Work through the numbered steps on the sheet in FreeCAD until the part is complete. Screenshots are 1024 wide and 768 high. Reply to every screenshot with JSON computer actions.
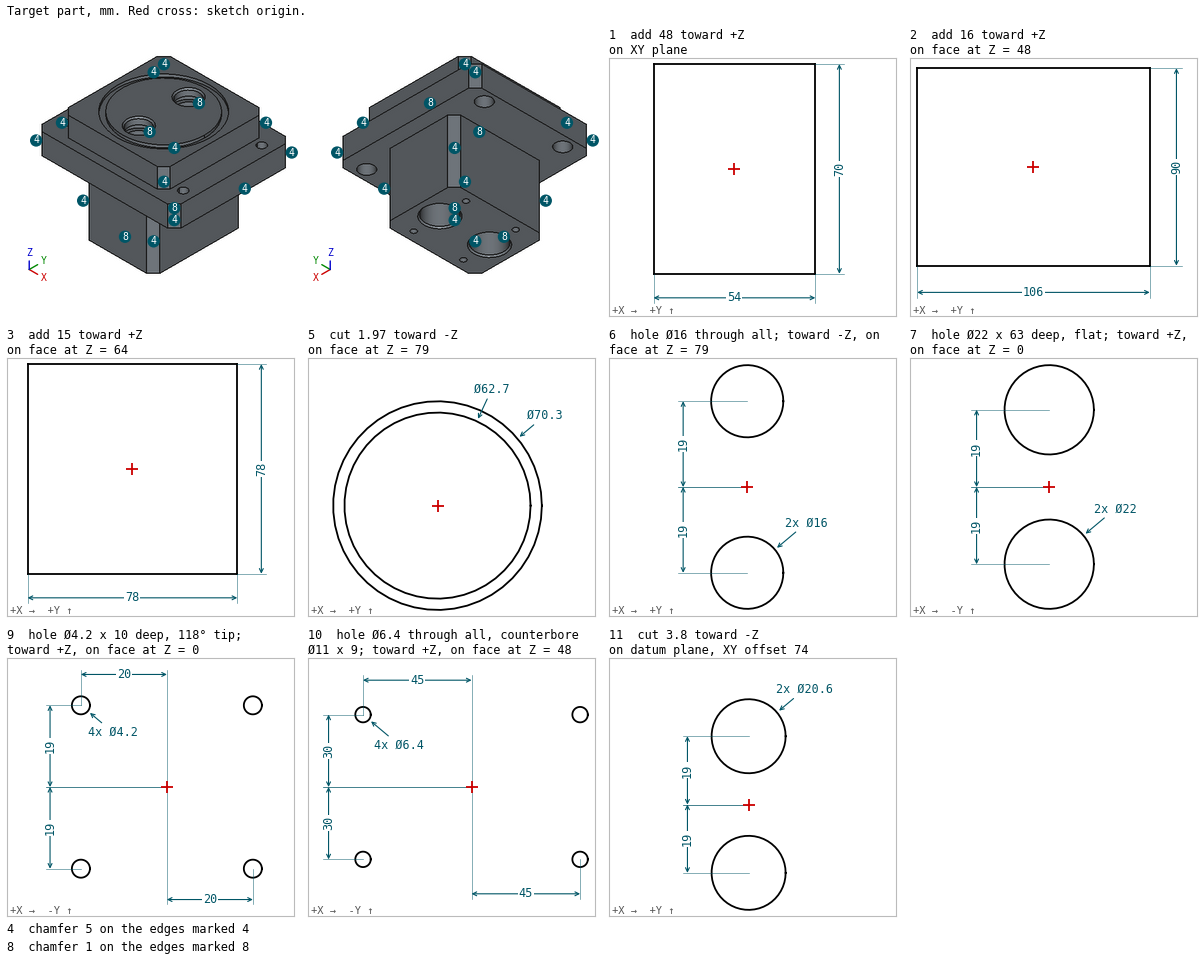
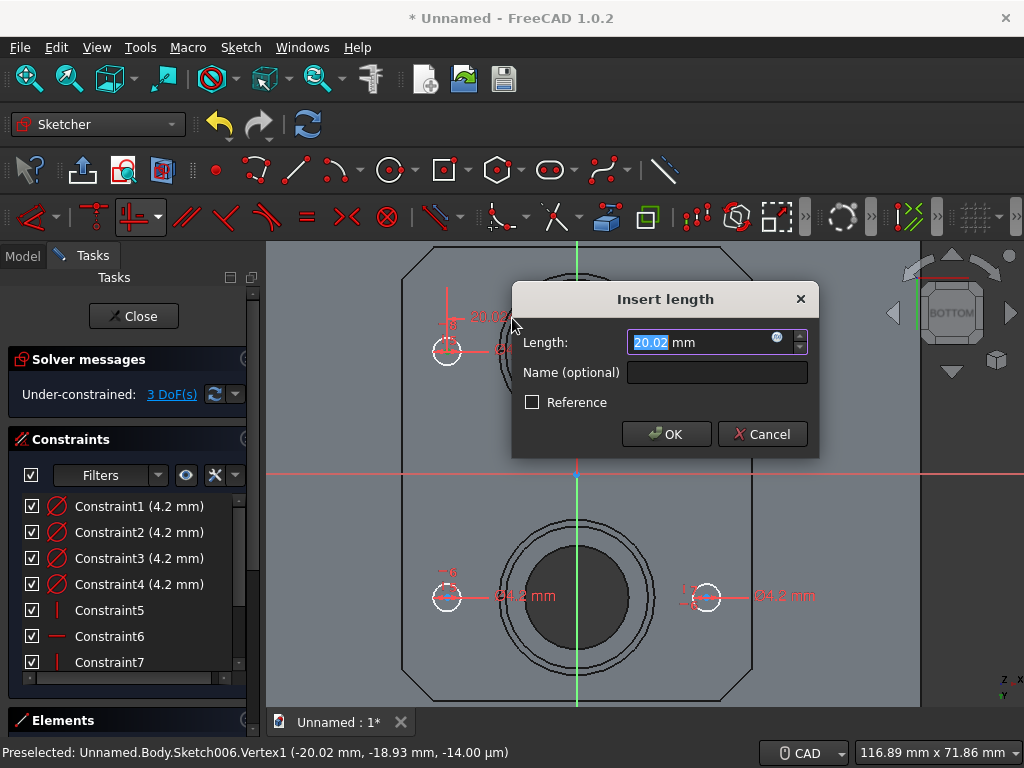
{"action": "type", "text": "20"}
{"action": "key", "text": "Return"}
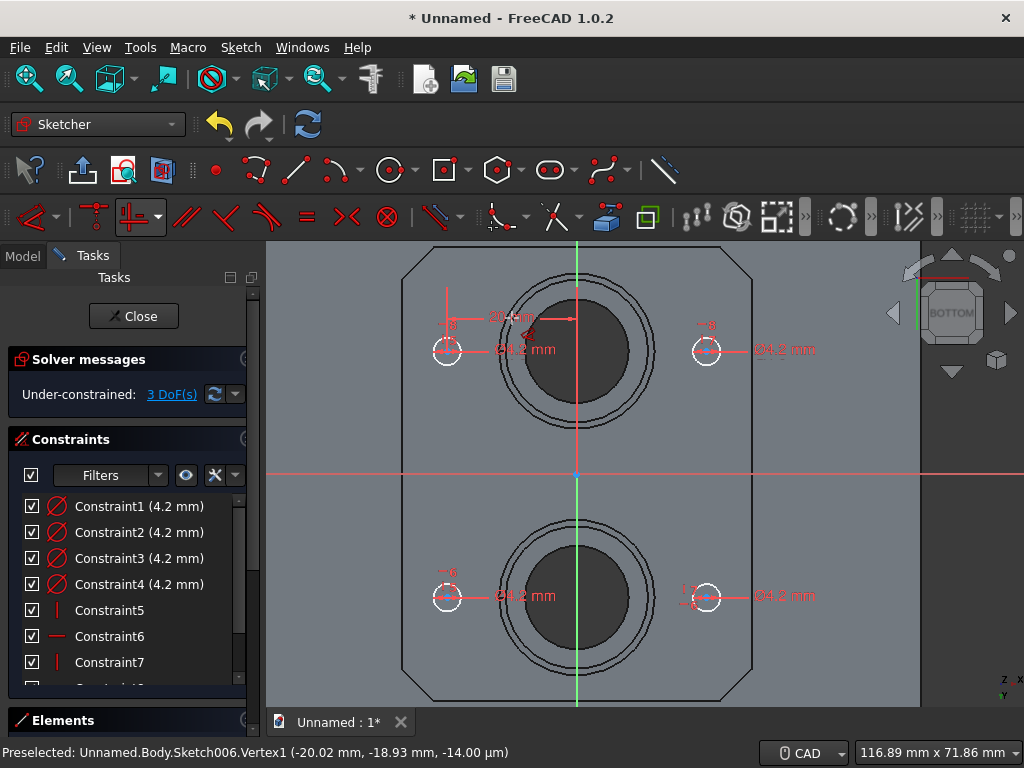
{"action": "left_click", "coordinate": [447, 352]}
{"action": "left_click", "coordinate": [413, 413]}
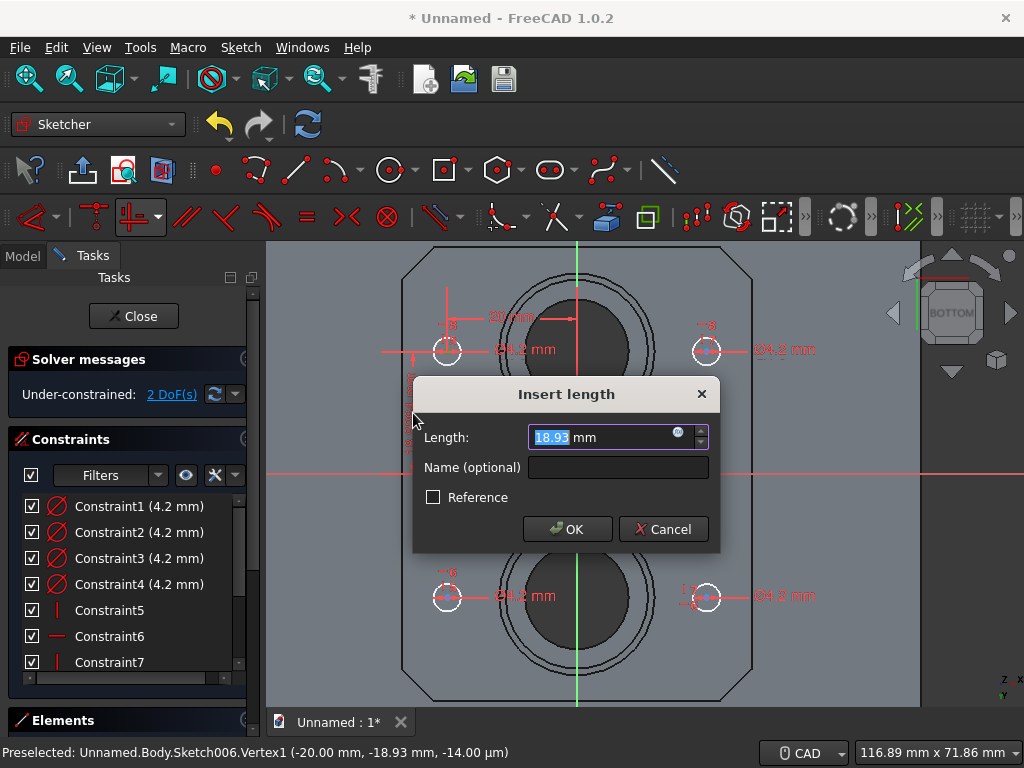
{"action": "type", "text": "19"}
{"action": "key", "text": "Return"}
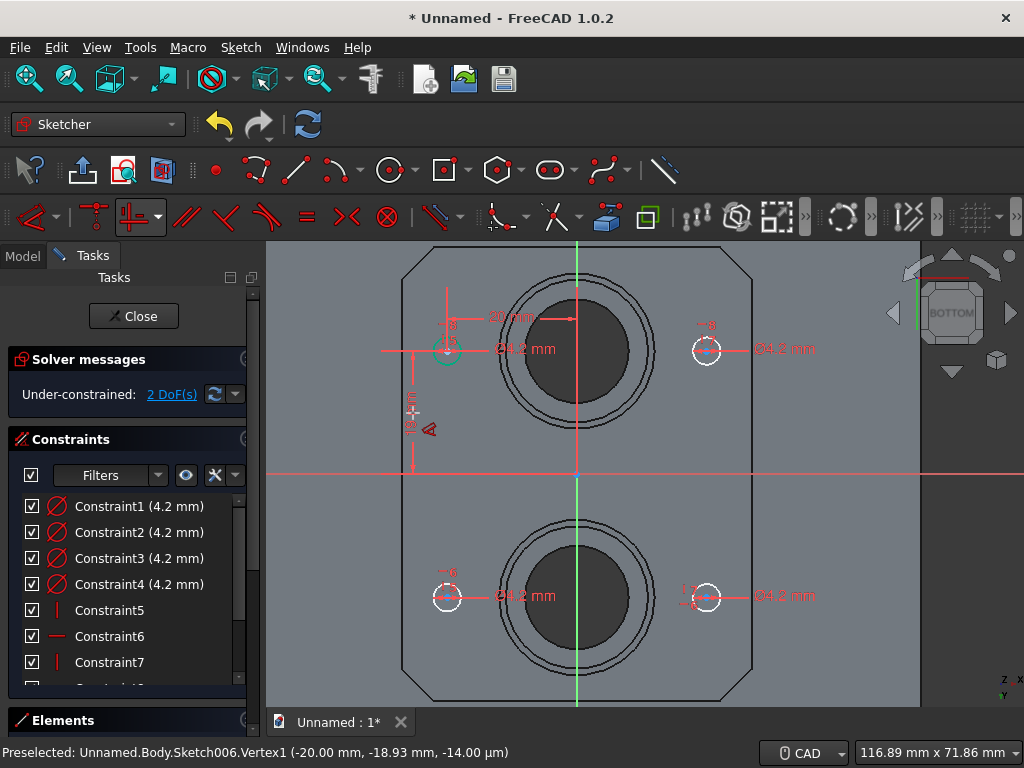
{"action": "left_click", "coordinate": [447, 598]}
{"action": "left_click", "coordinate": [413, 536]}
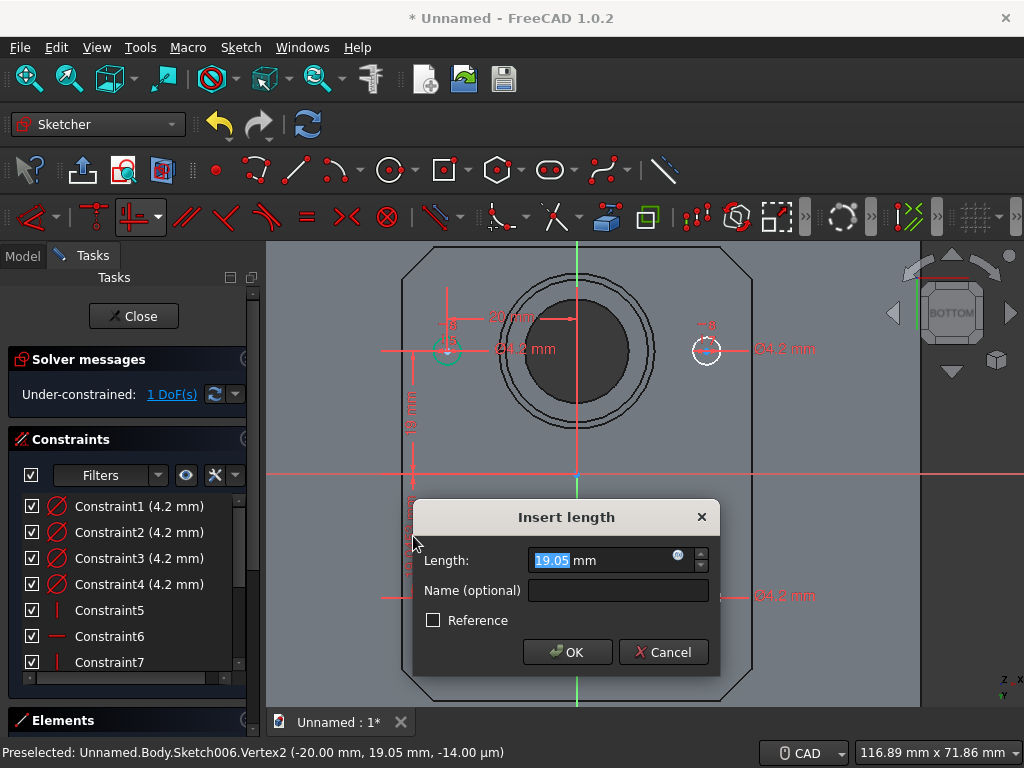
{"action": "type", "text": "19"}
{"action": "key", "text": "Return"}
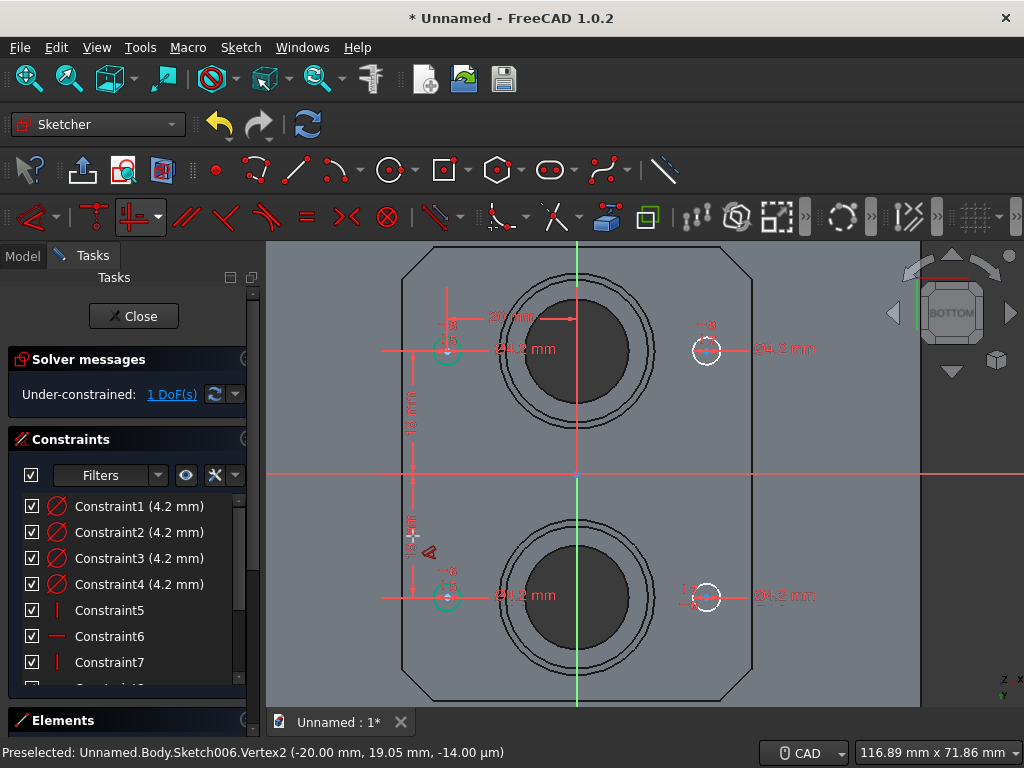
{"action": "left_click", "coordinate": [707, 598]}
{"action": "left_click", "coordinate": [642, 632]}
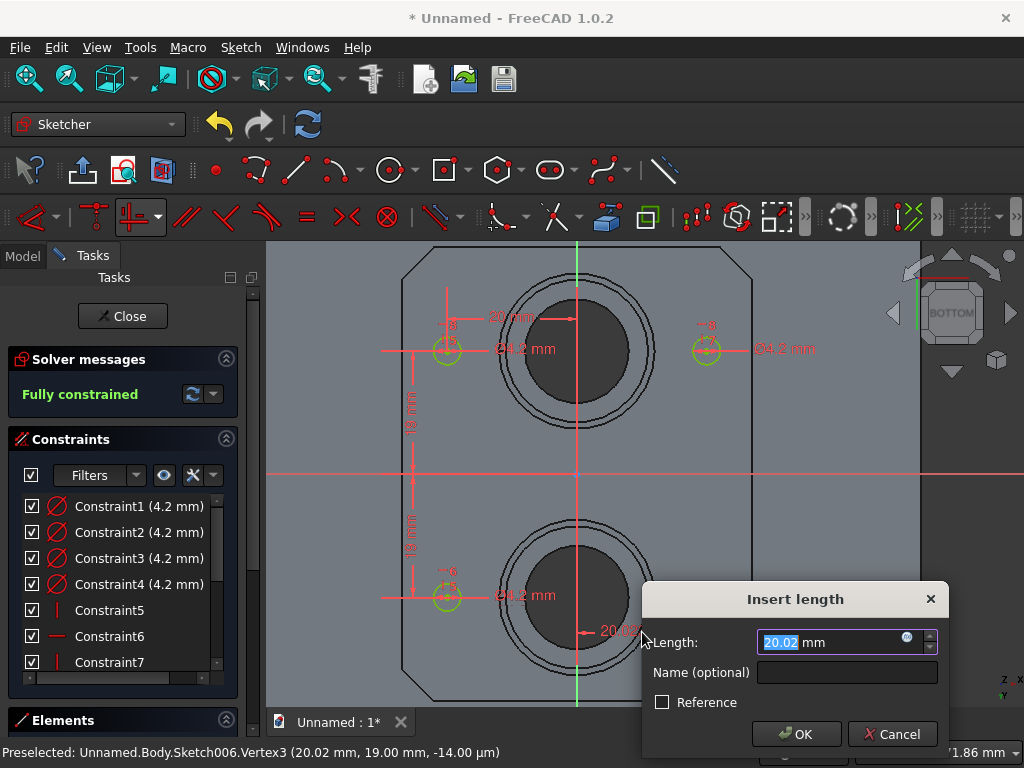
{"action": "type", "text": "20"}
{"action": "key", "text": "Return"}
{"action": "key", "text": "Escape"}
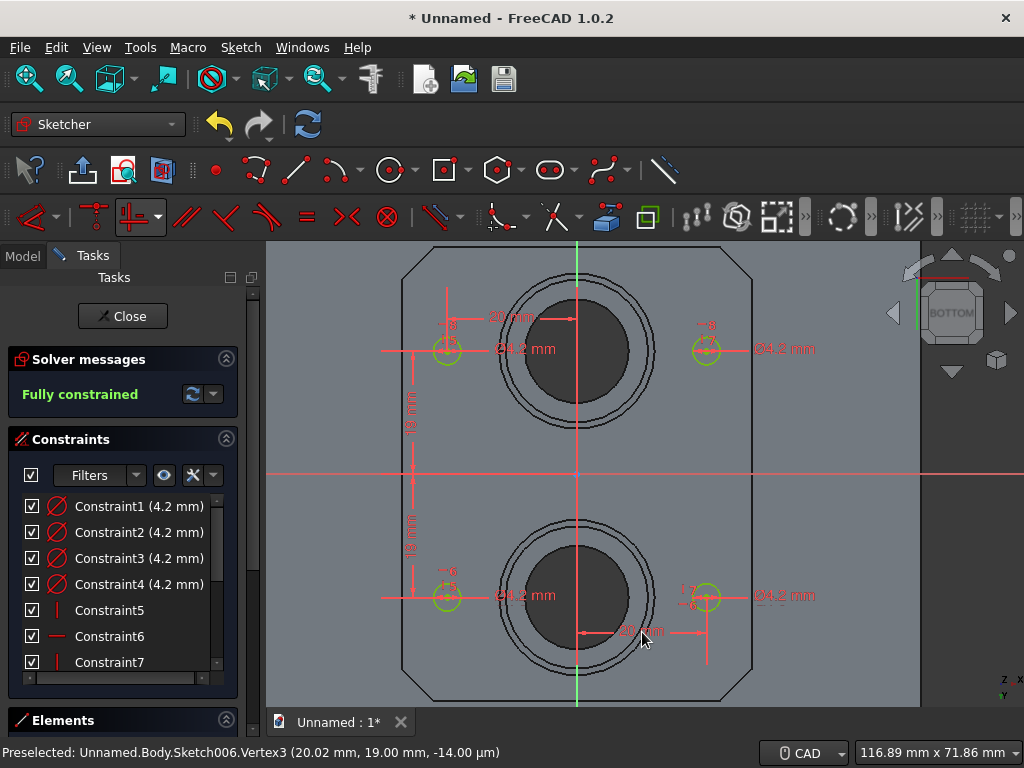
{"action": "left_click", "coordinate": [123, 316]}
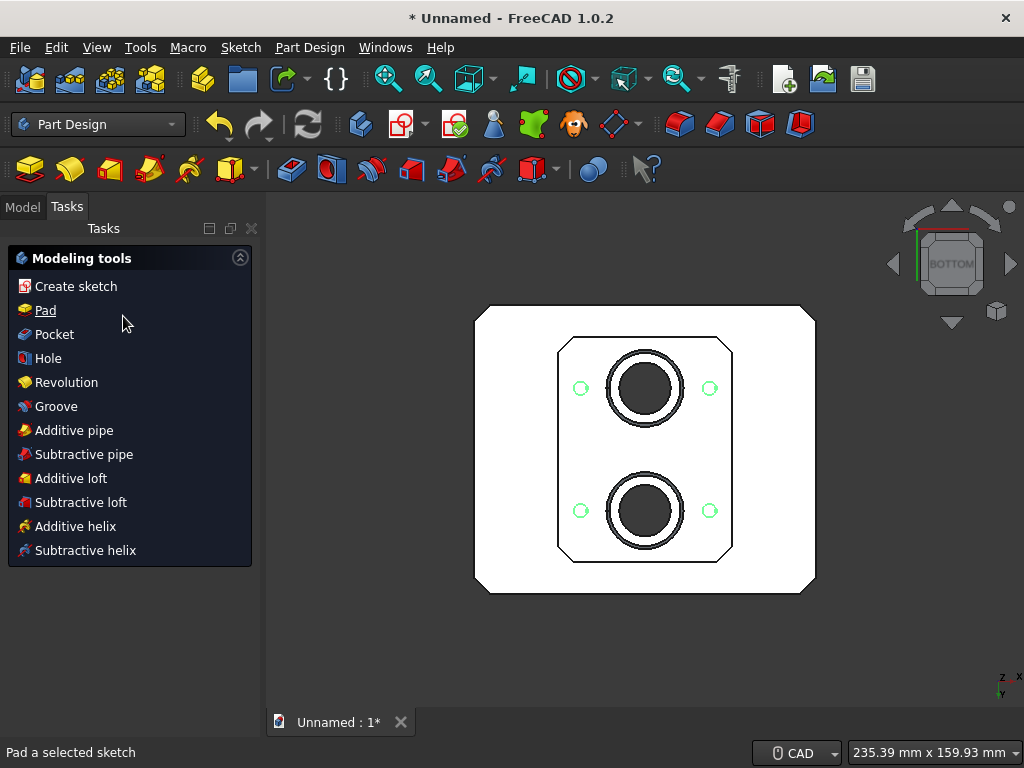
{"action": "left_click", "coordinate": [332, 170]}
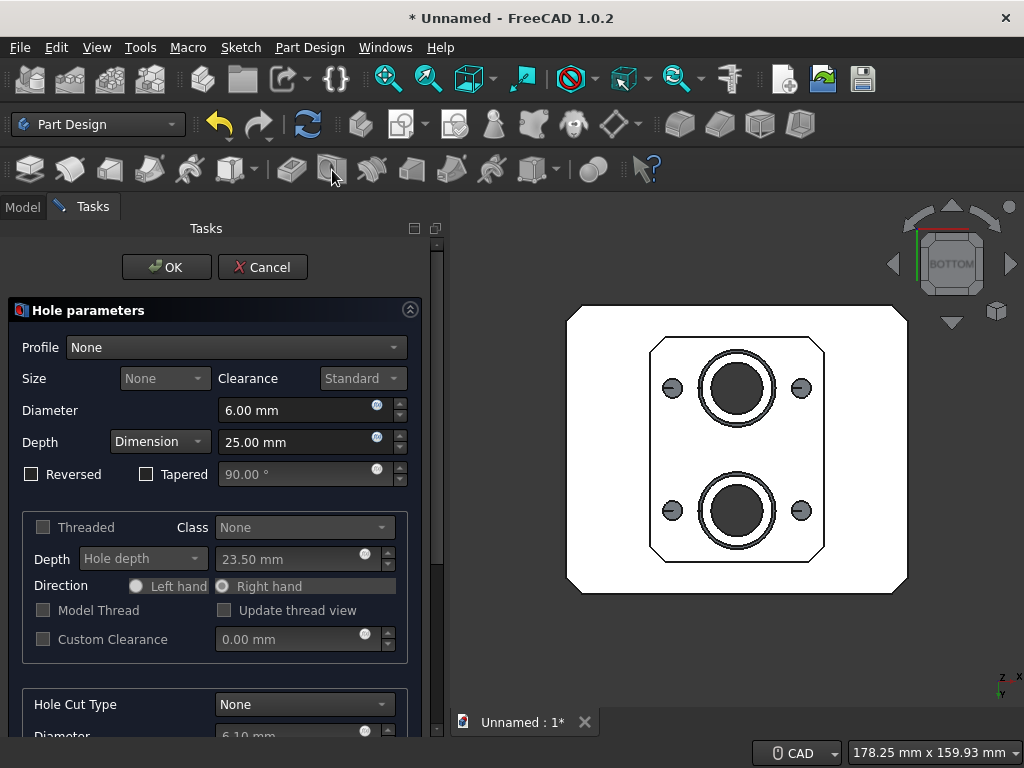
{"action": "triple_click", "coordinate": [305, 410]}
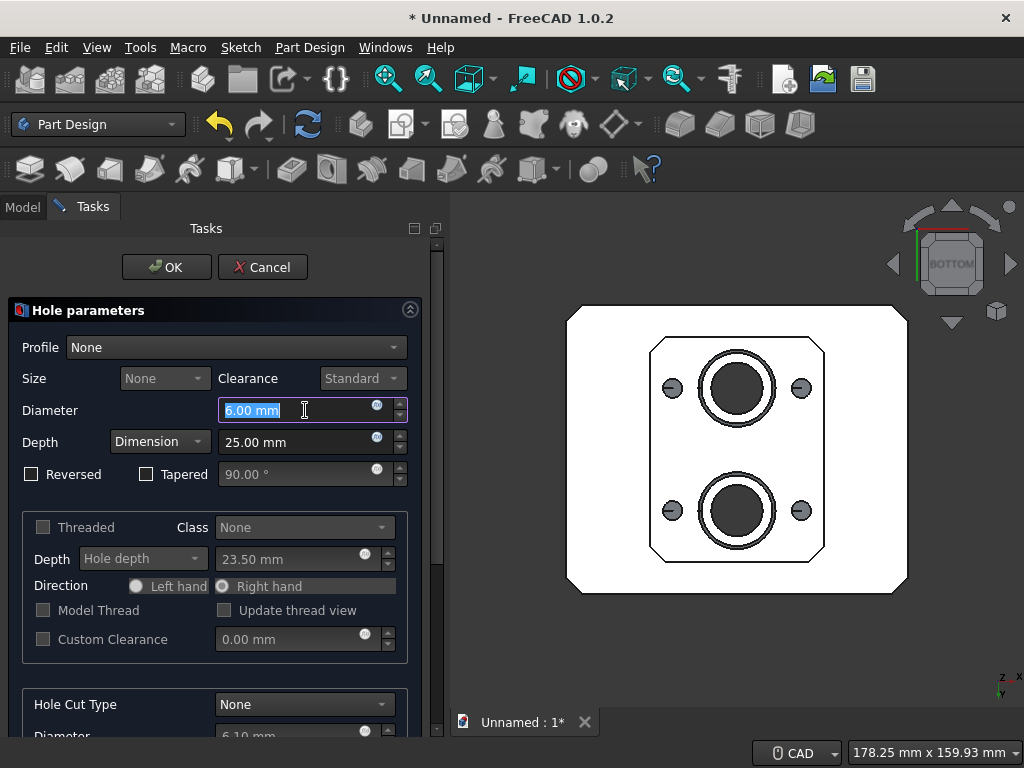
{"action": "type", "text": "4.2"}
{"action": "key", "text": "Tab"}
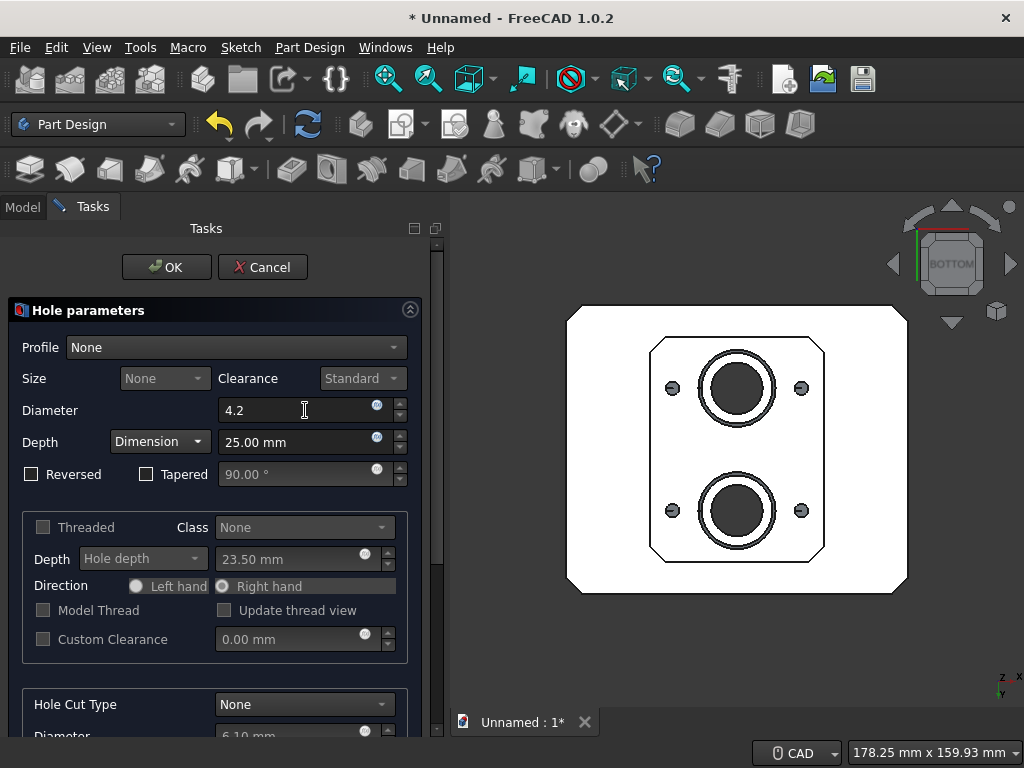
{"action": "triple_click", "coordinate": [305, 442]}